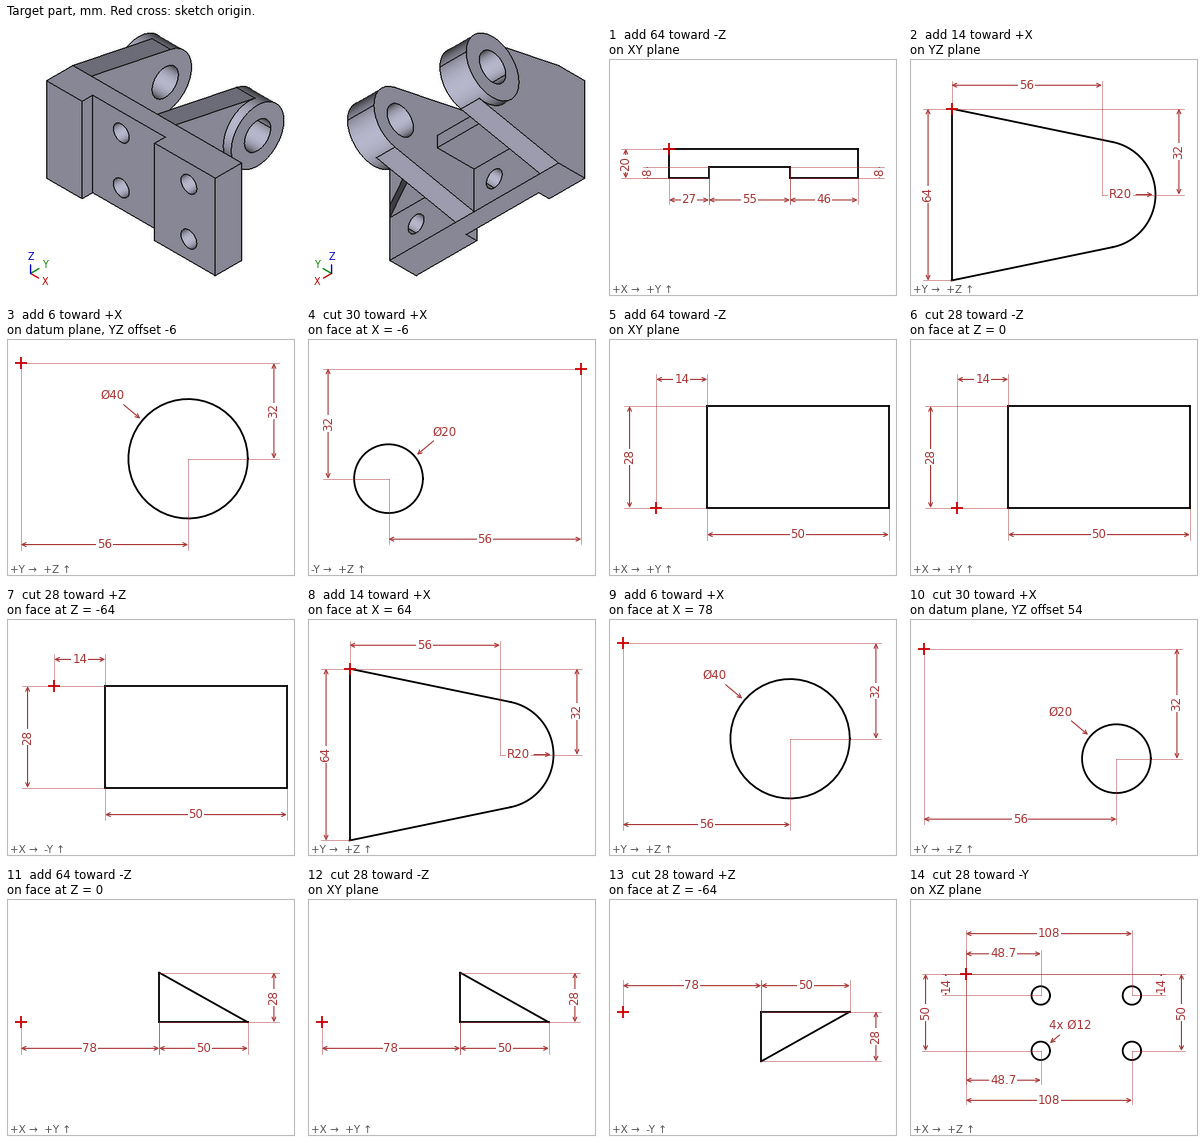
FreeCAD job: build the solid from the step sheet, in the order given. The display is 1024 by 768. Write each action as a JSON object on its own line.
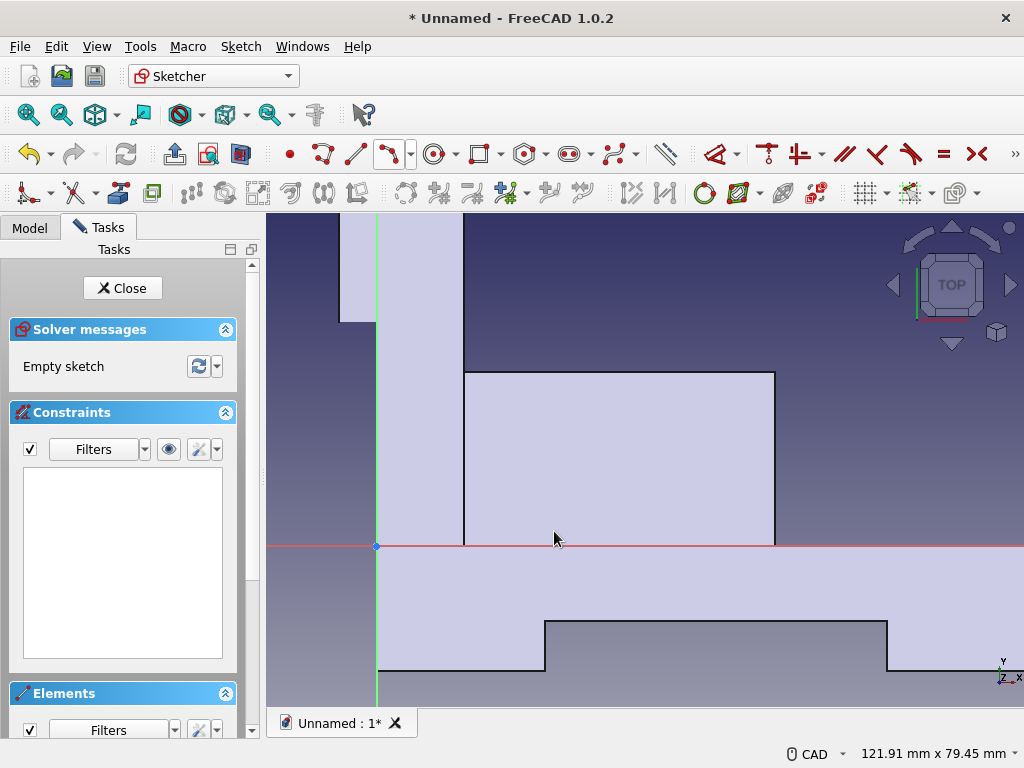
{"action": "left_click", "coordinate": [478, 154]}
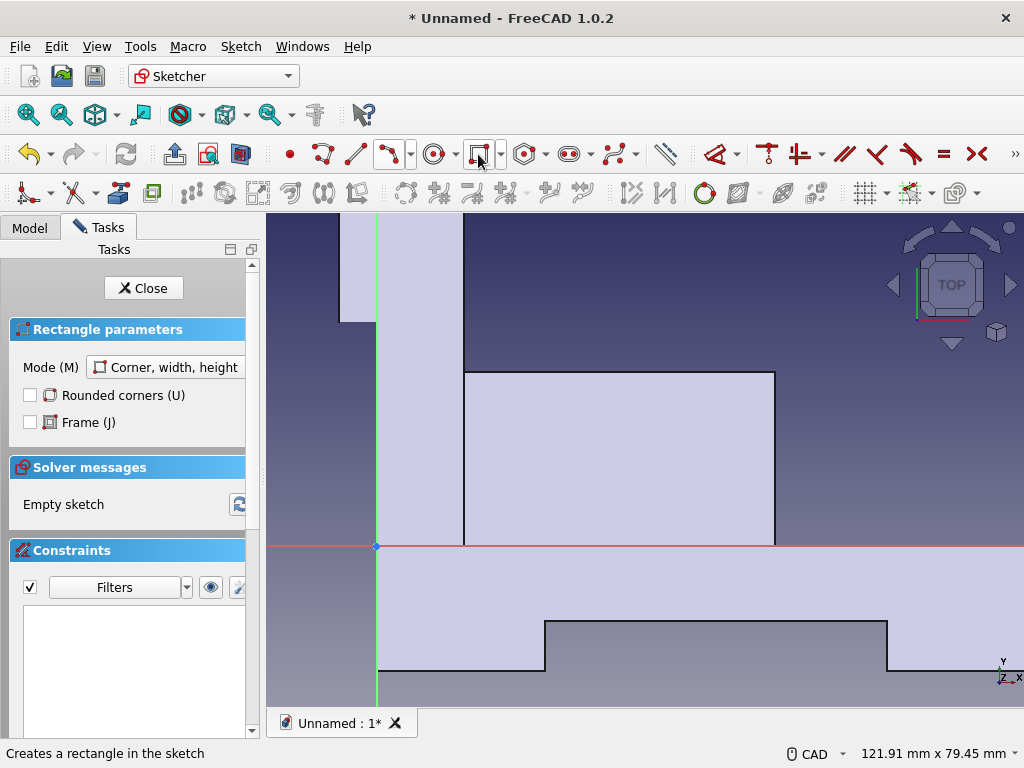
{"action": "left_click", "coordinate": [464, 372]}
{"action": "left_click", "coordinate": [775, 546]}
{"action": "key", "text": "Escape"}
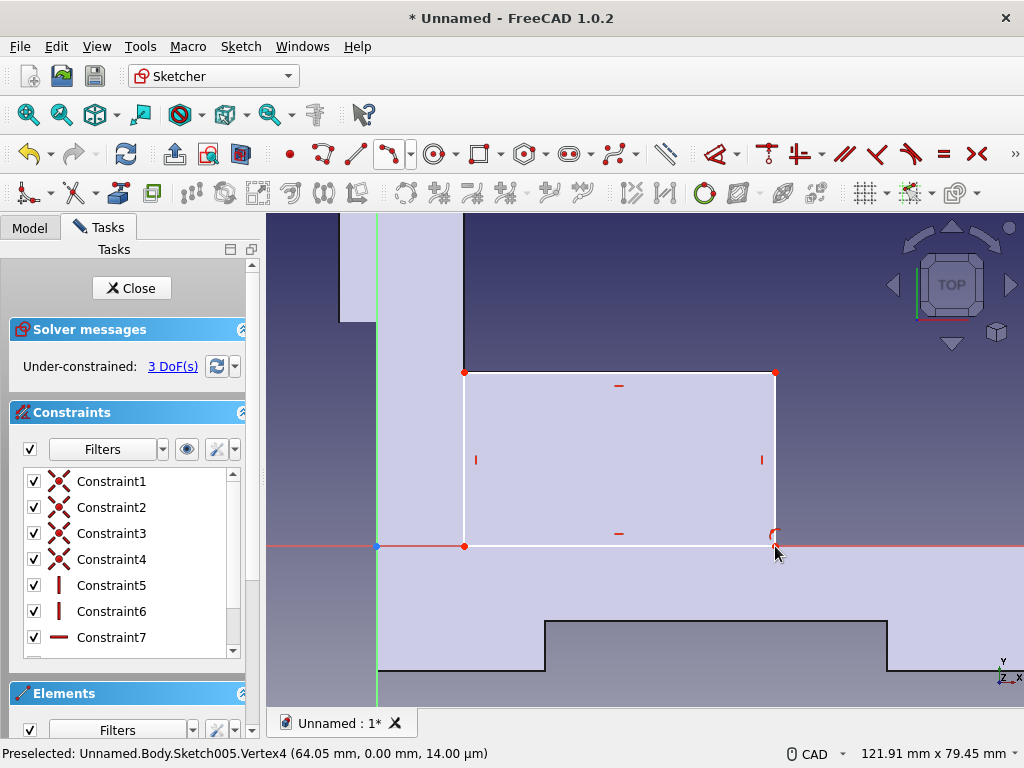
{"action": "left_click", "coordinate": [714, 154]}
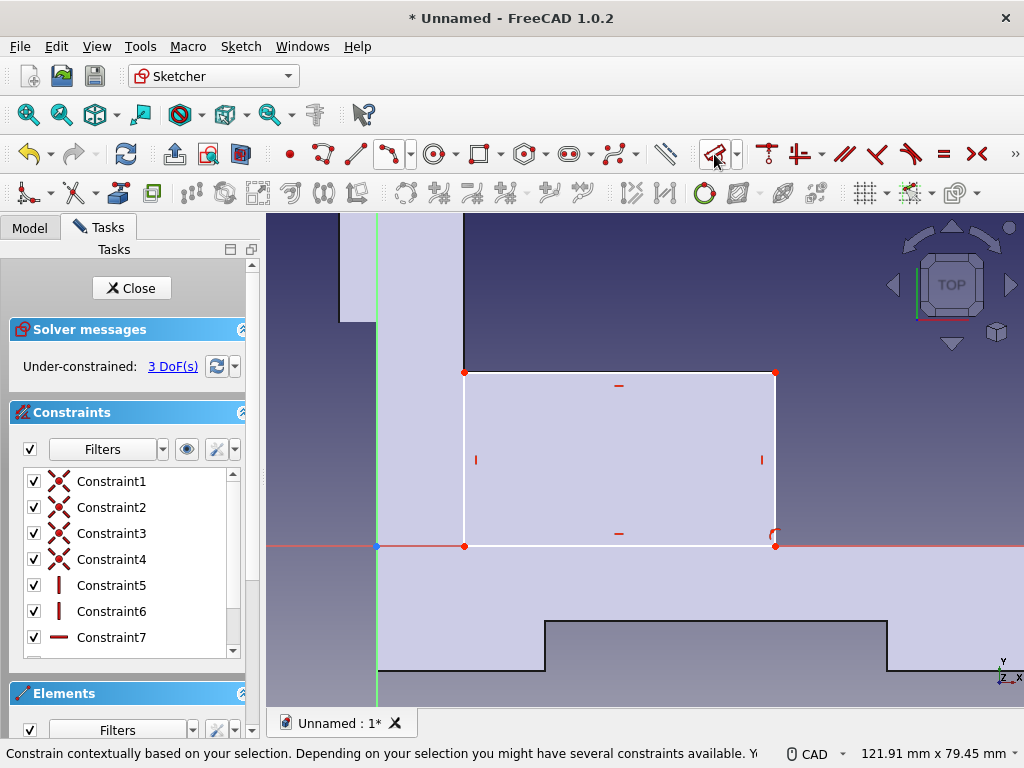
{"action": "left_click", "coordinate": [464, 425]}
{"action": "left_click", "coordinate": [430, 460]}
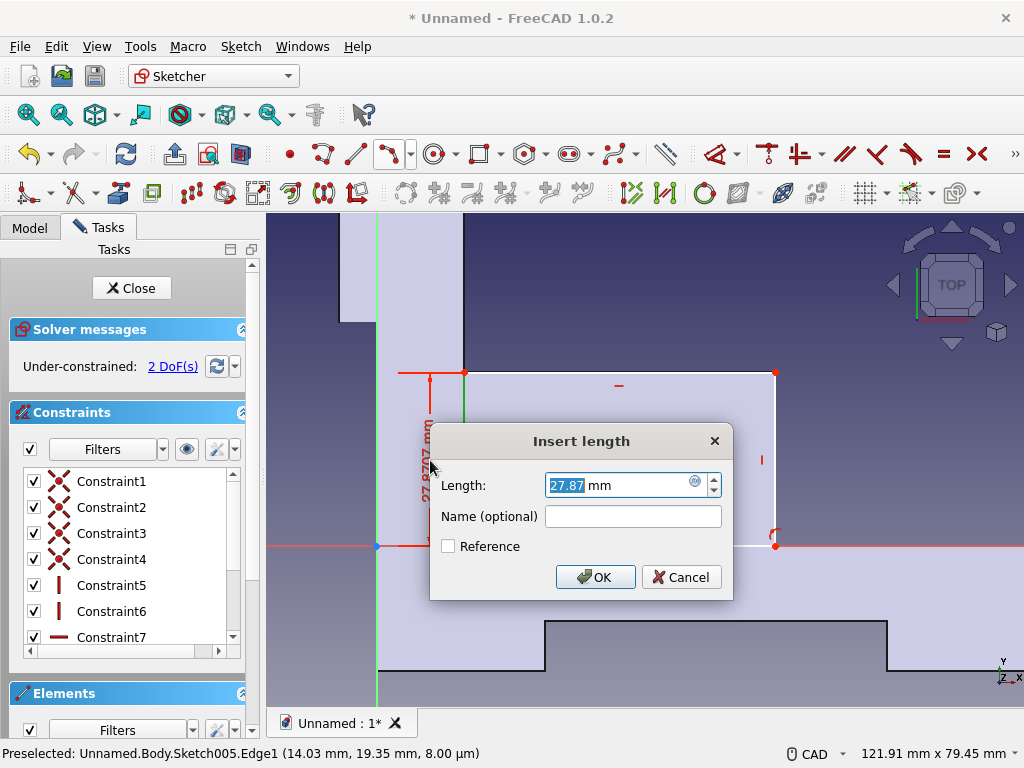
{"action": "type", "text": "28"}
{"action": "key", "text": "Return"}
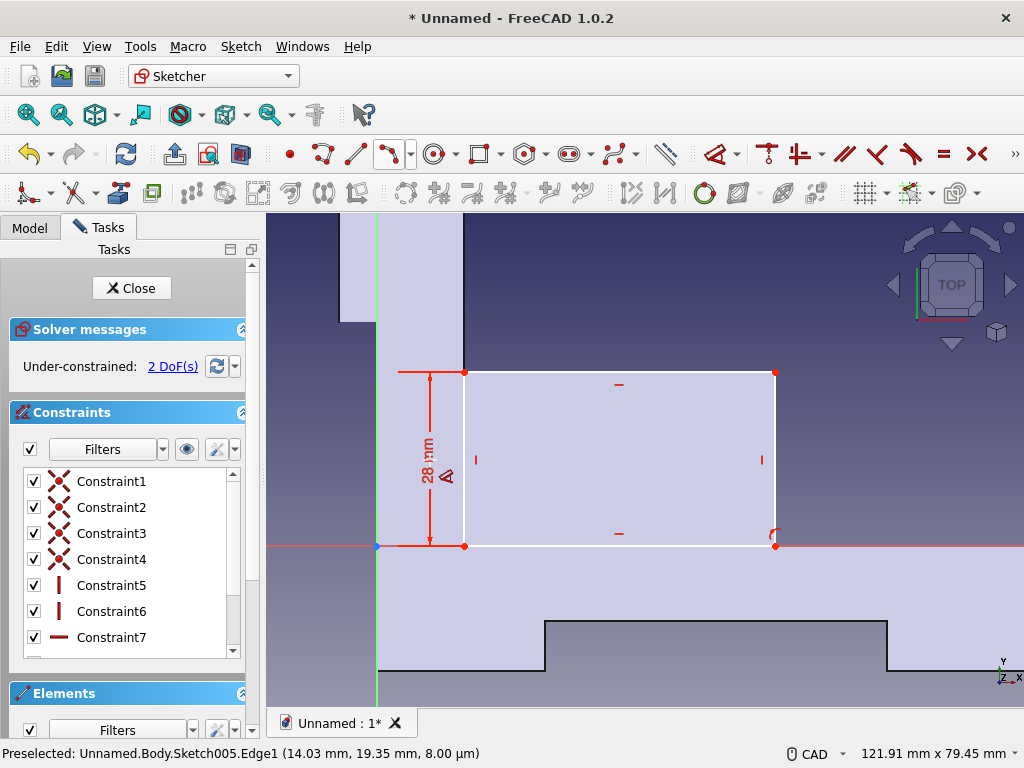
{"action": "left_click", "coordinate": [557, 546]}
{"action": "left_click", "coordinate": [620, 580]}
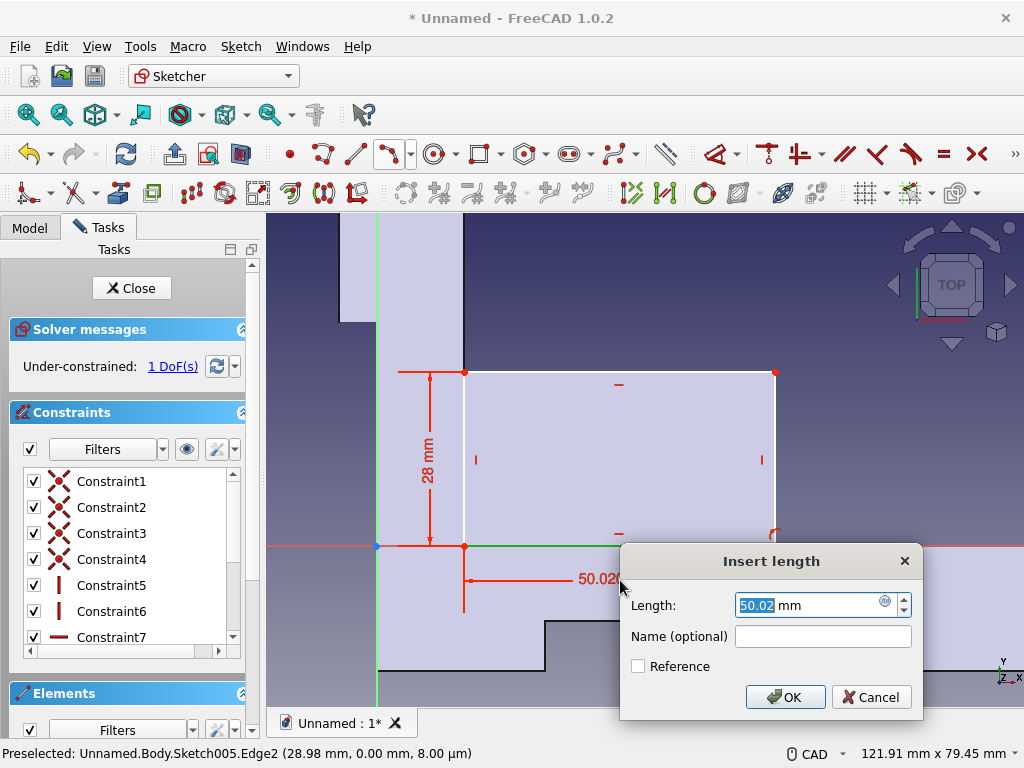
{"action": "type", "text": "50"}
{"action": "key", "text": "Return"}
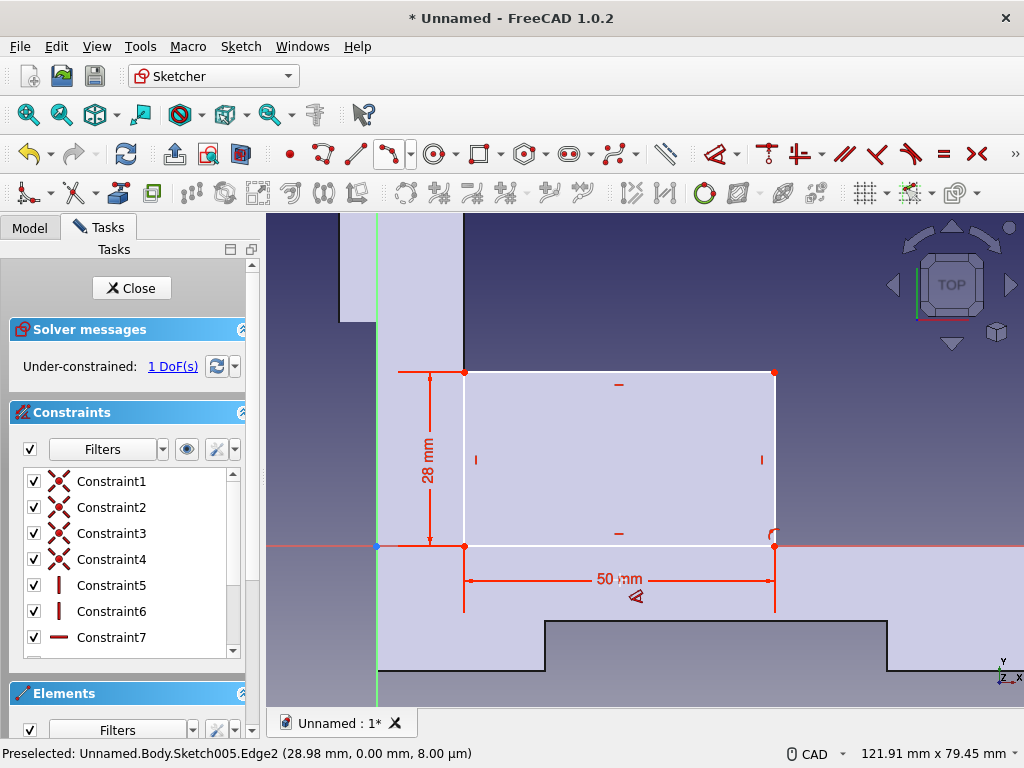
{"action": "left_click", "coordinate": [464, 372]}
{"action": "left_click", "coordinate": [420, 580]}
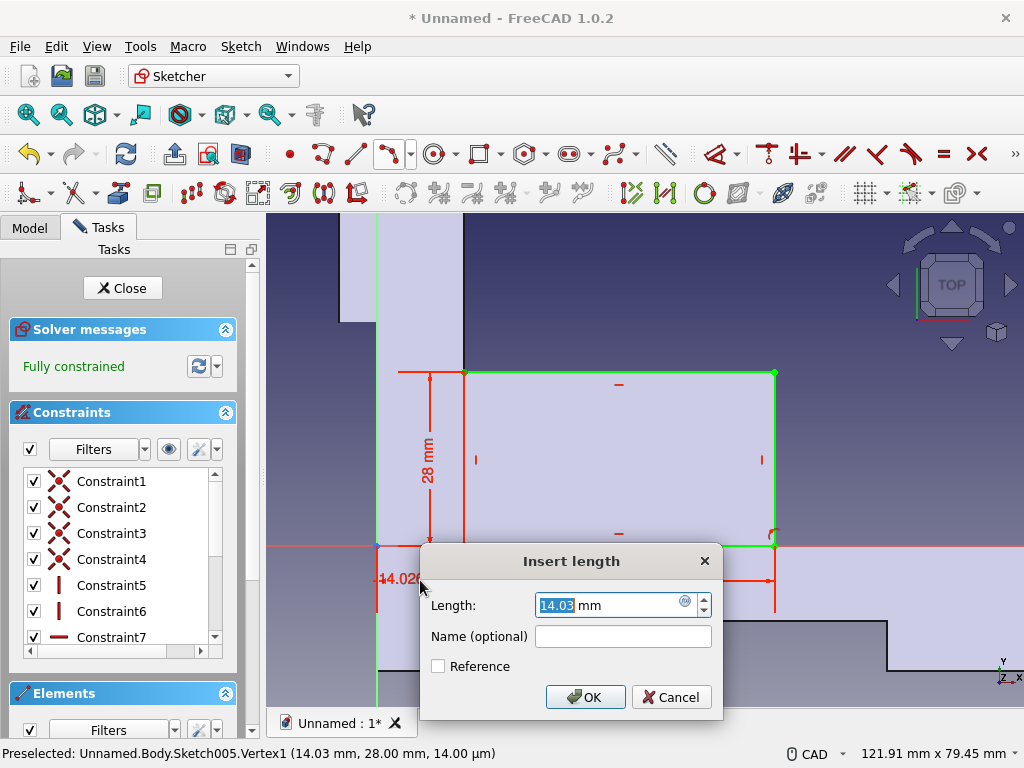
{"action": "type", "text": "14"}
{"action": "key", "text": "Return"}
{"action": "key", "text": "Escape"}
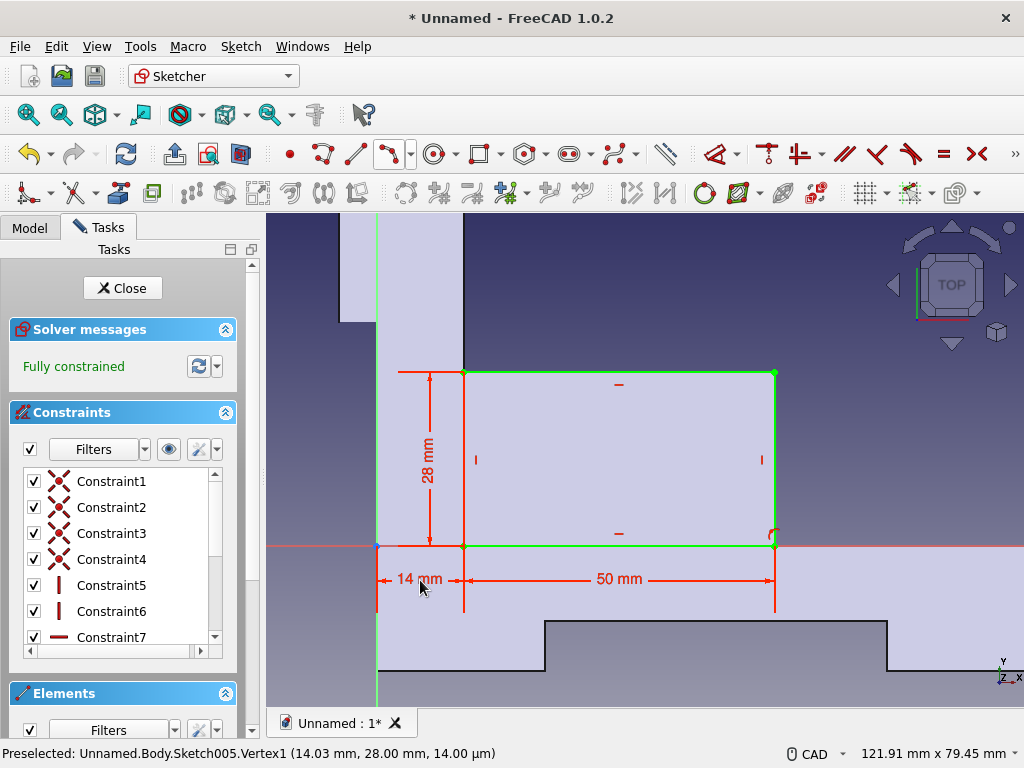
{"action": "left_click", "coordinate": [123, 288]}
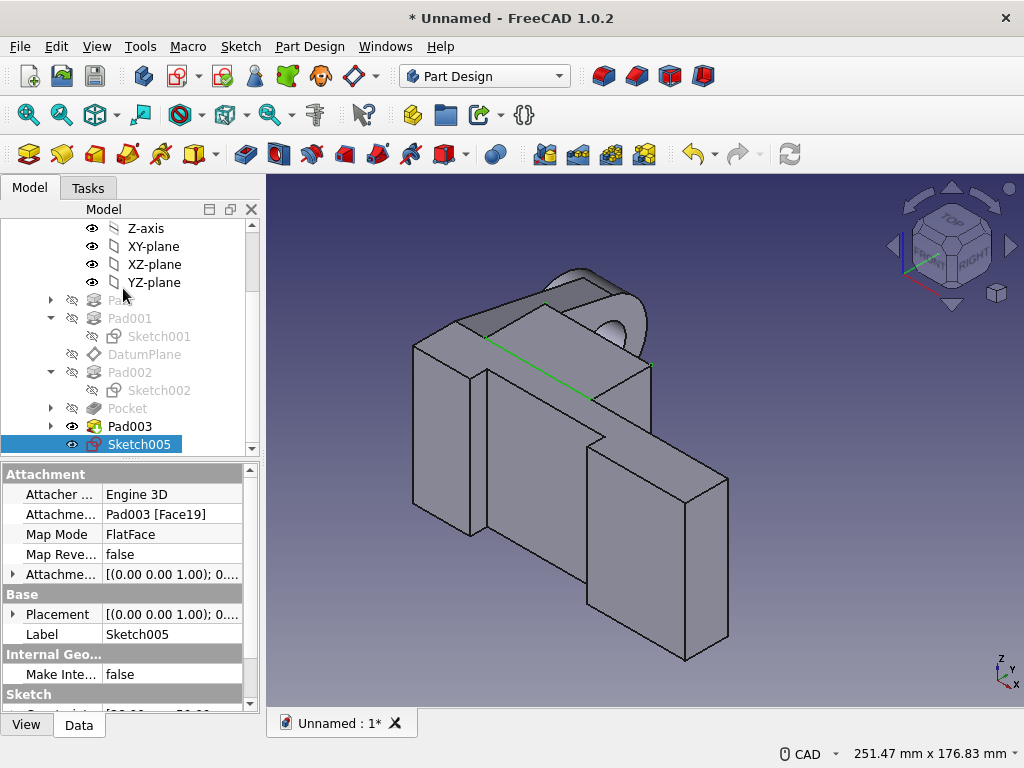
{"action": "left_click", "coordinate": [246, 154]}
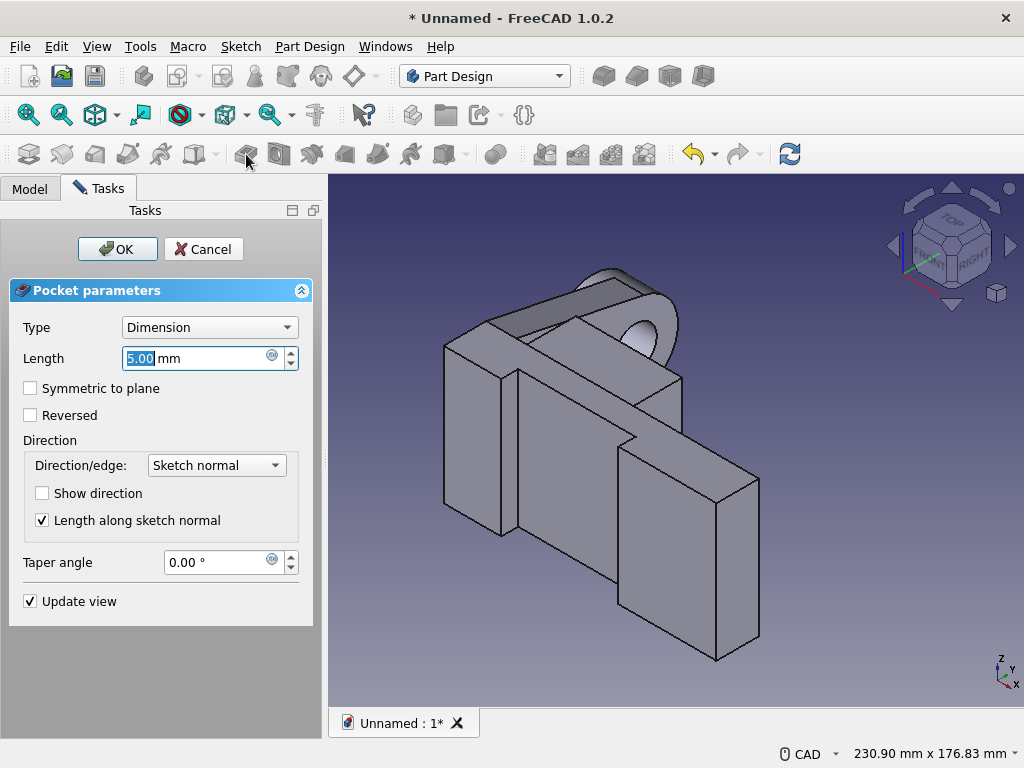
{"action": "type", "text": "28"}
{"action": "key", "text": "Tab"}